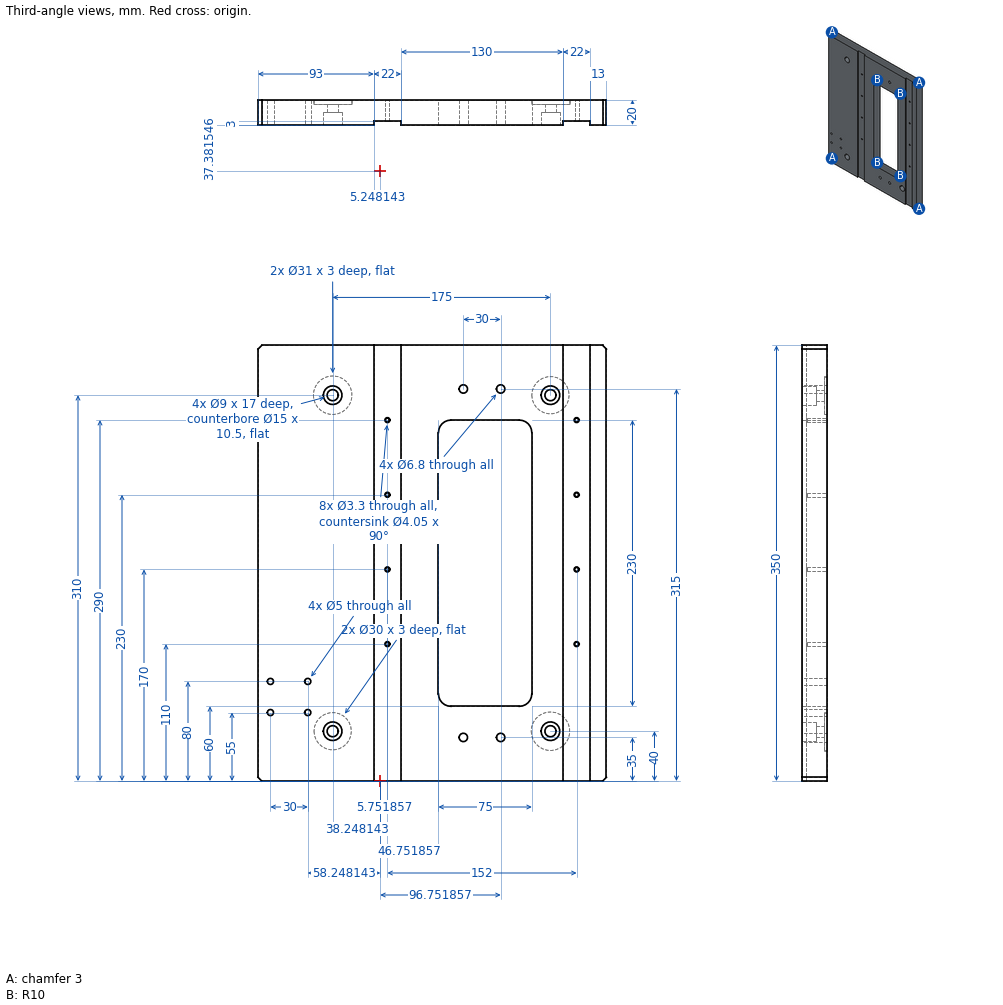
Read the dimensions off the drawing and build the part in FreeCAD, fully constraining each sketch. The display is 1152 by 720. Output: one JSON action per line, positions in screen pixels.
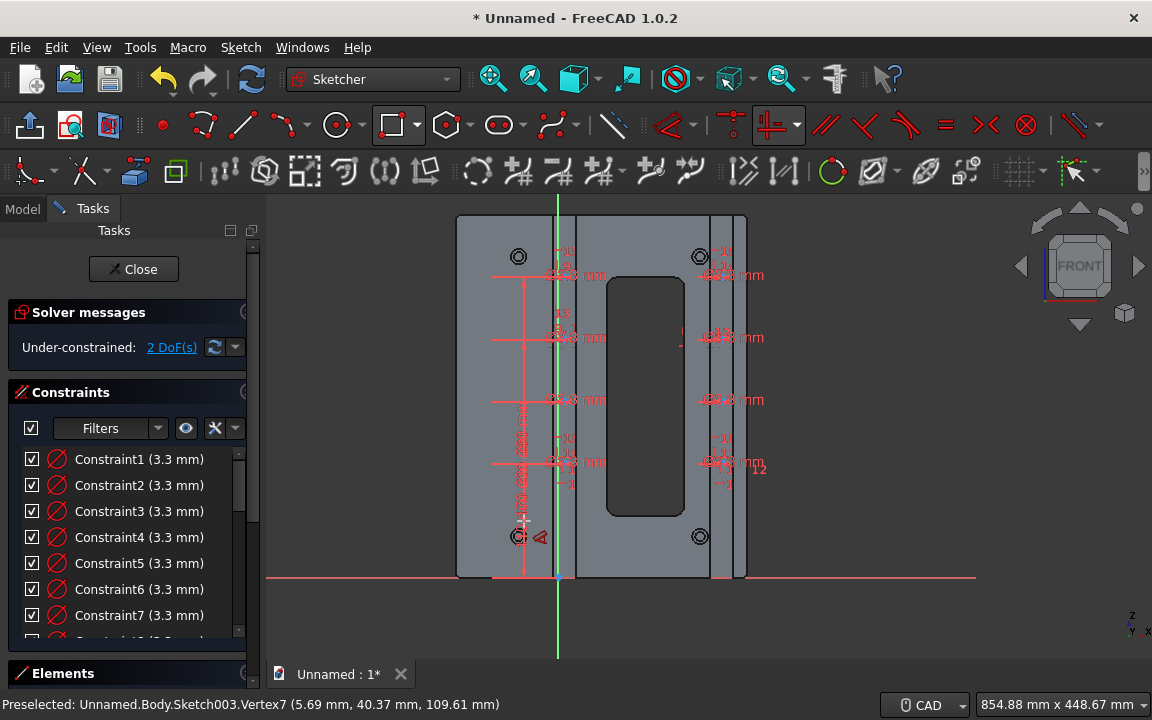
{"action": "left_click", "coordinate": [564, 402]}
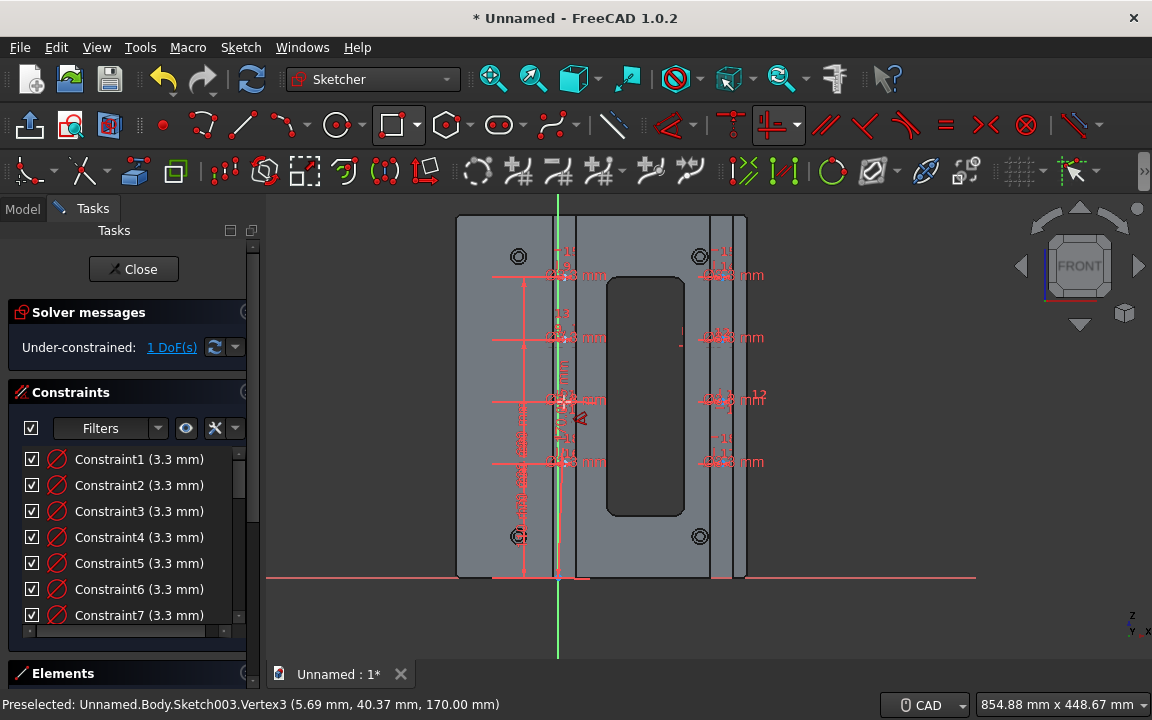
{"action": "left_click", "coordinate": [722, 402]}
{"action": "left_click", "coordinate": [643, 368]}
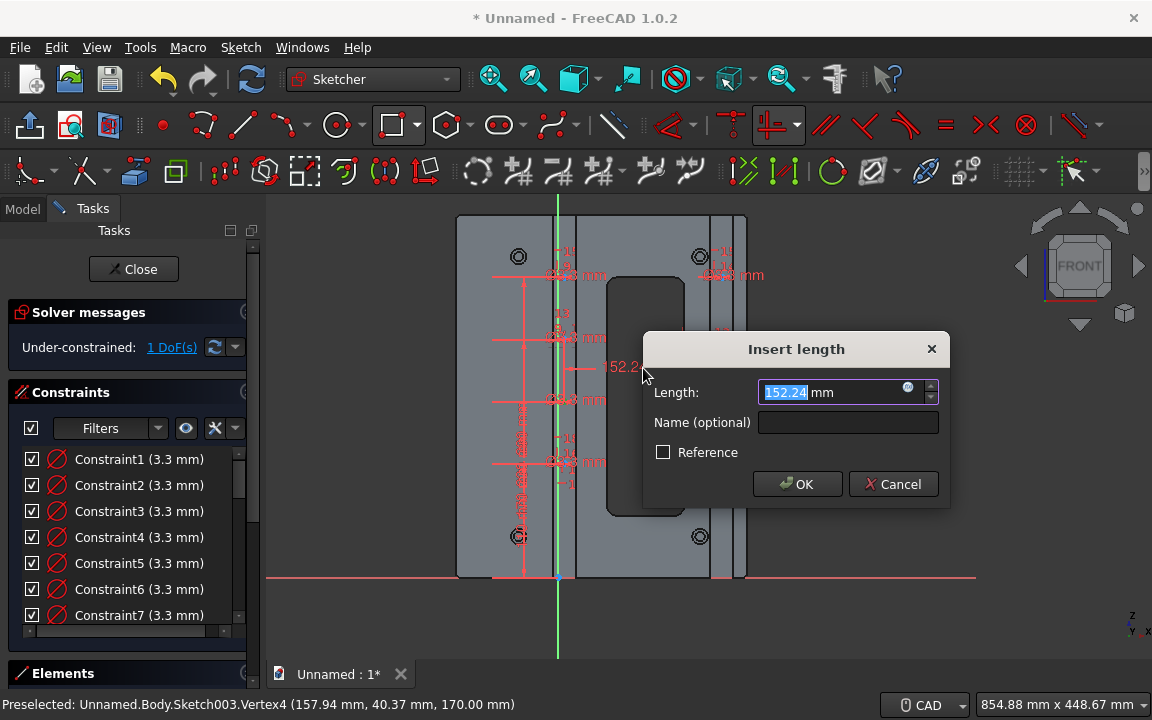
{"action": "type", "text": "152"}
{"action": "key", "text": "Return"}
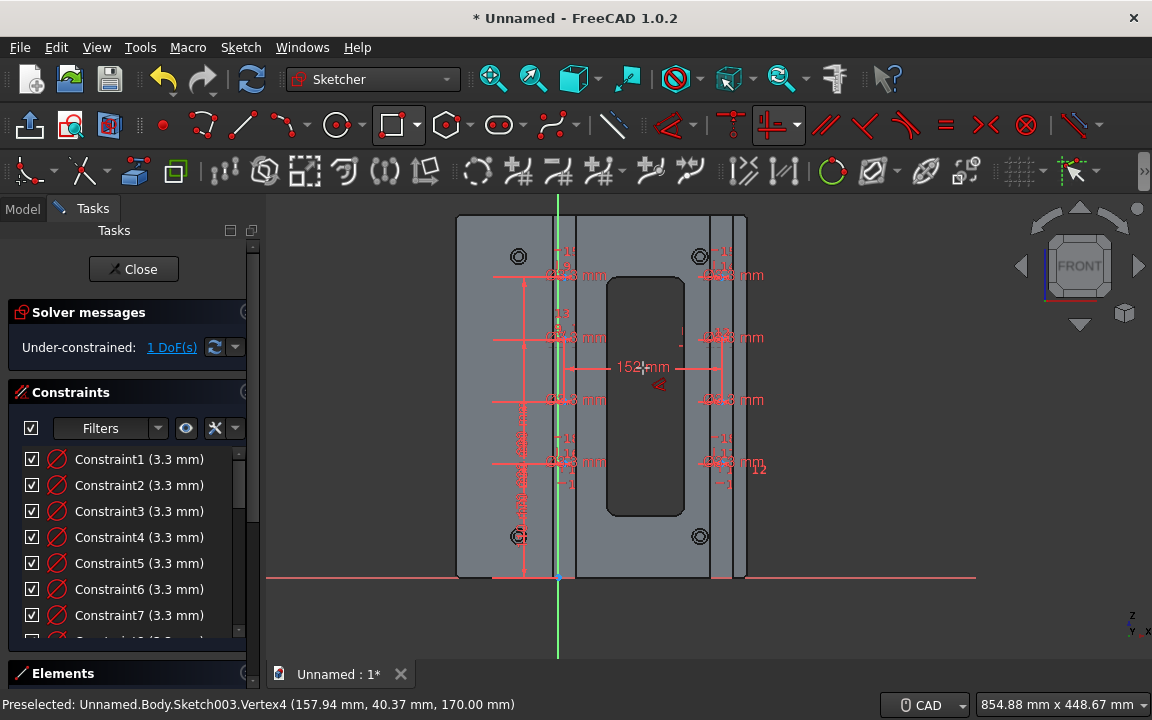
{"action": "scroll", "coordinate": [564, 277], "scroll_direction": "up", "scroll_amount": 10}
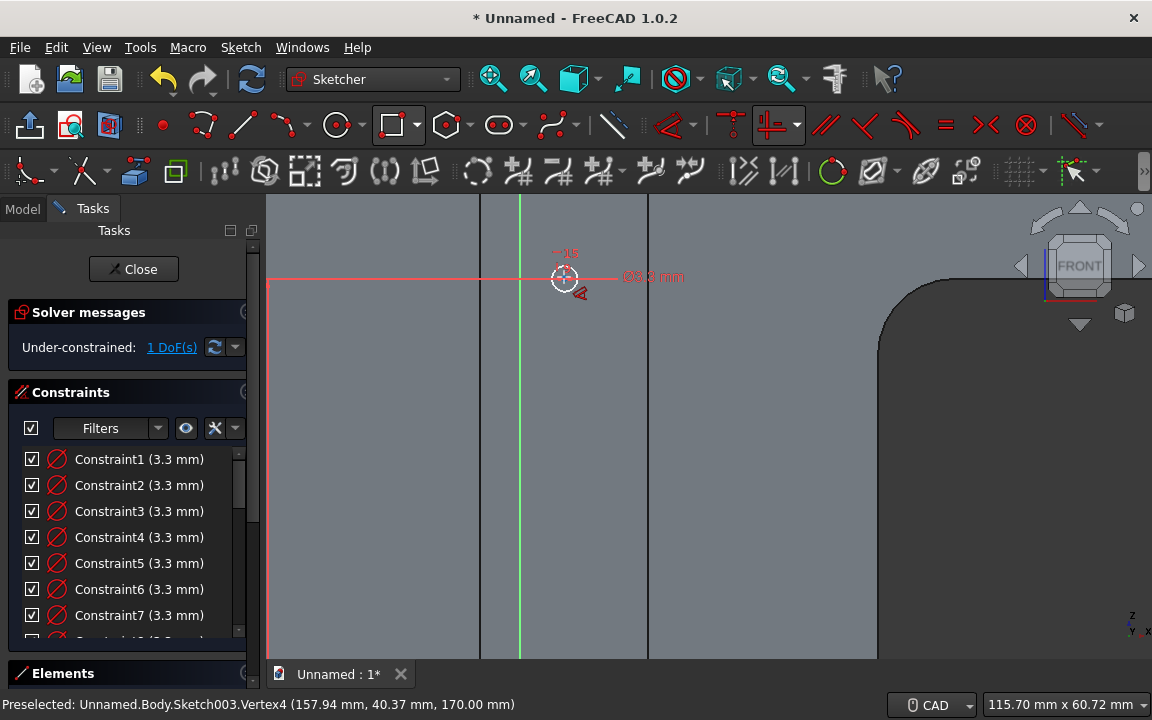
{"action": "left_click", "coordinate": [565, 279]}
{"action": "left_click", "coordinate": [542, 245]}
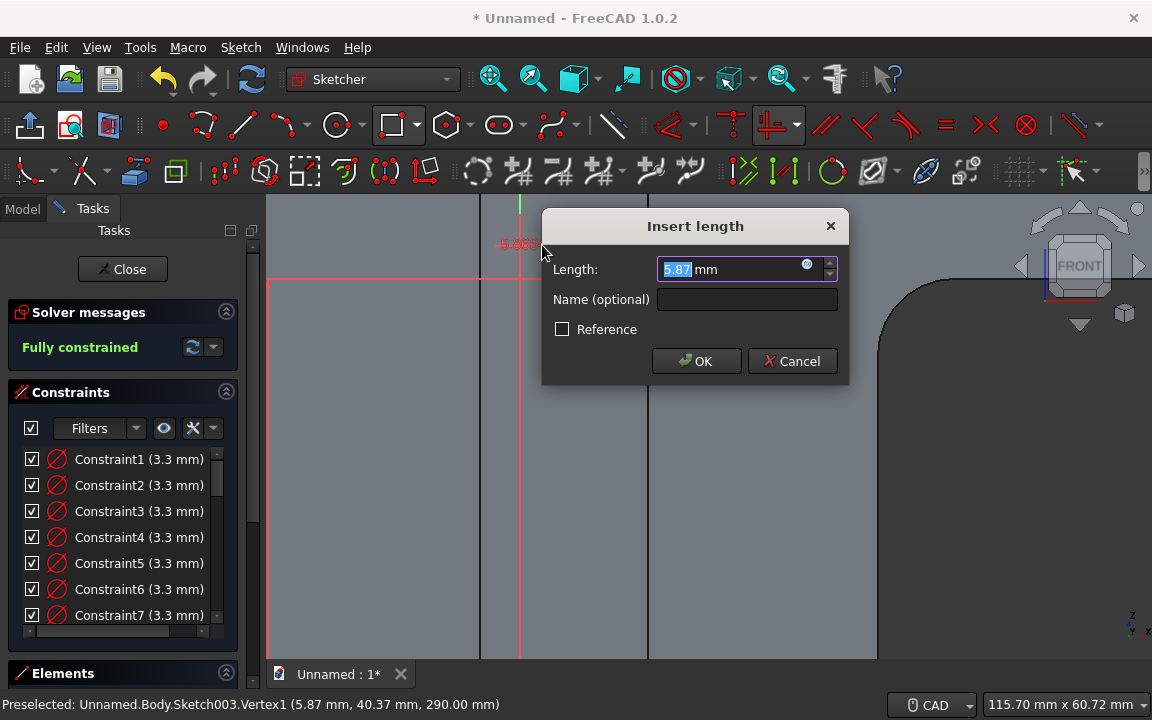
{"action": "type", "text": "5.751857"}
{"action": "key", "text": "Return"}
{"action": "key", "text": "Escape"}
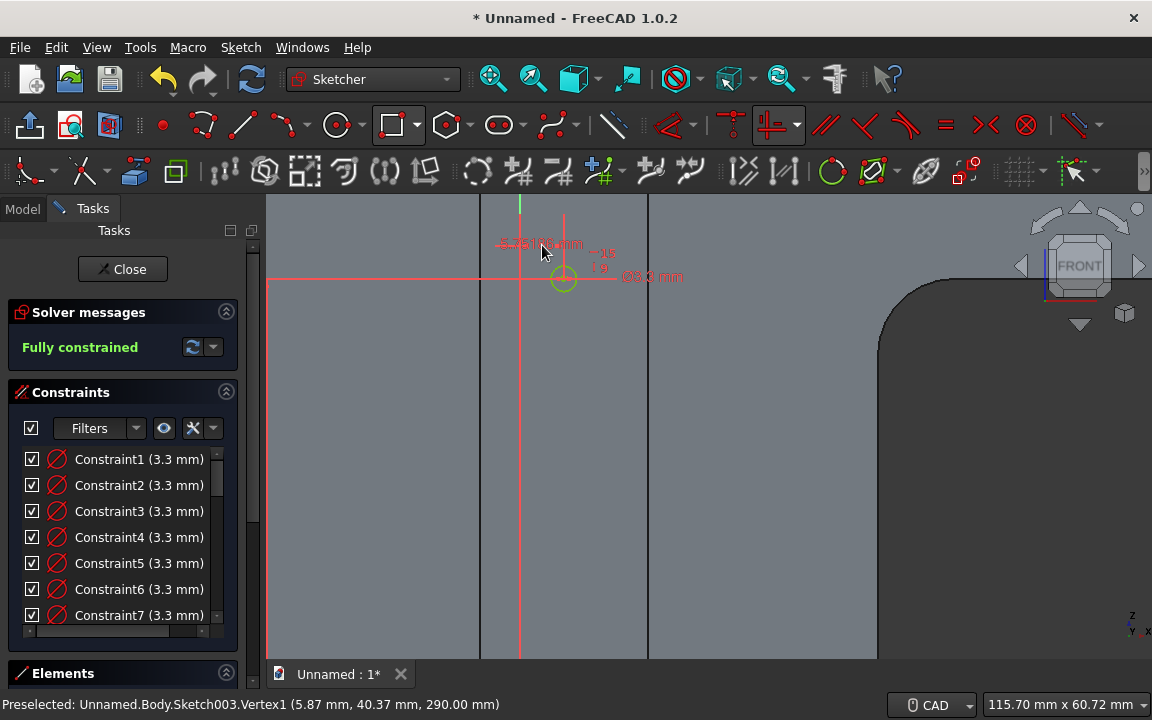
{"action": "left_click", "coordinate": [123, 269]}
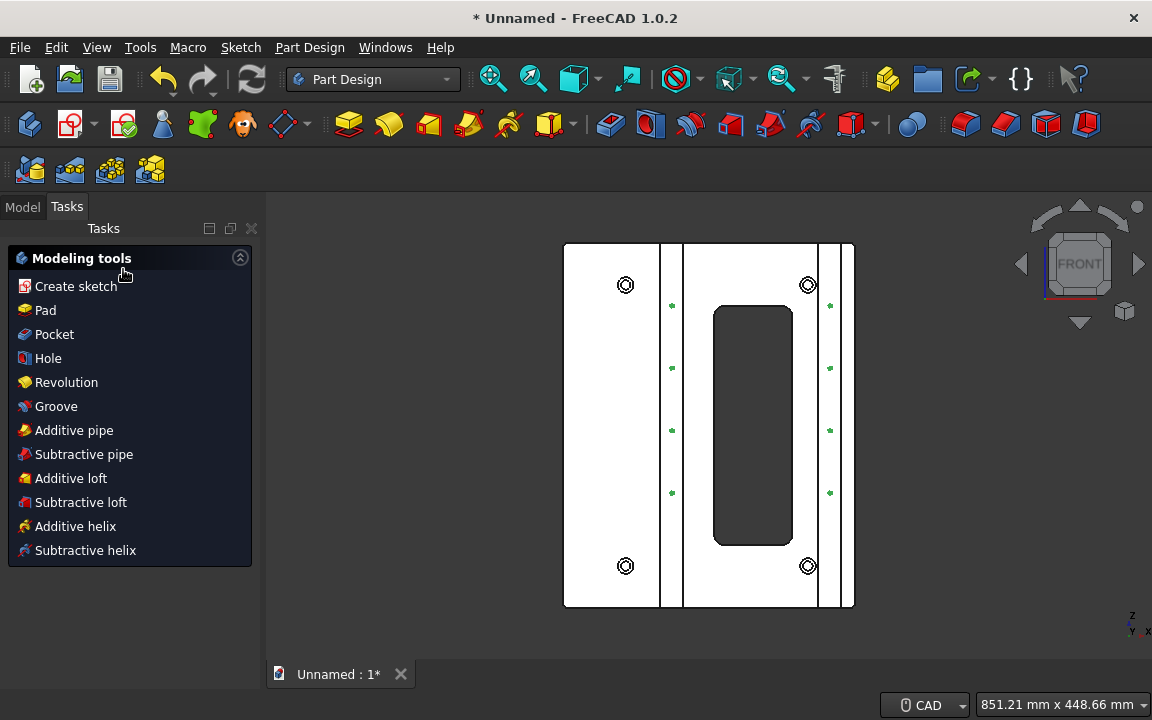
{"action": "left_click", "coordinate": [652, 124]}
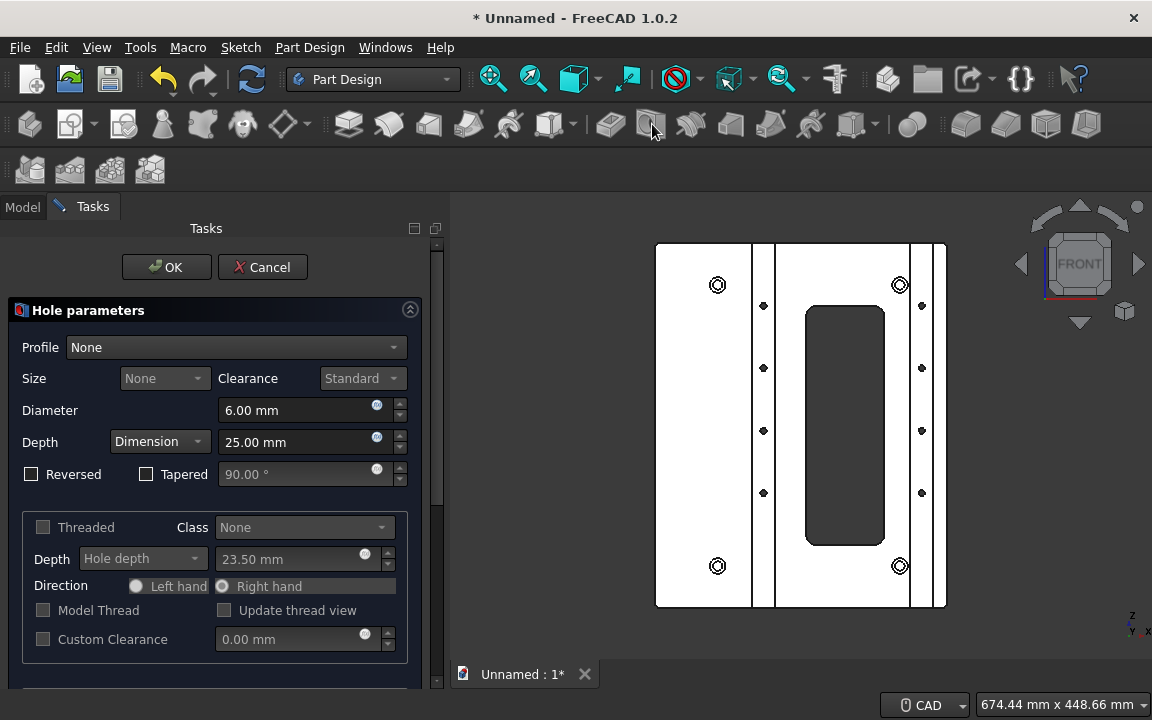
{"action": "triple_click", "coordinate": [305, 410]}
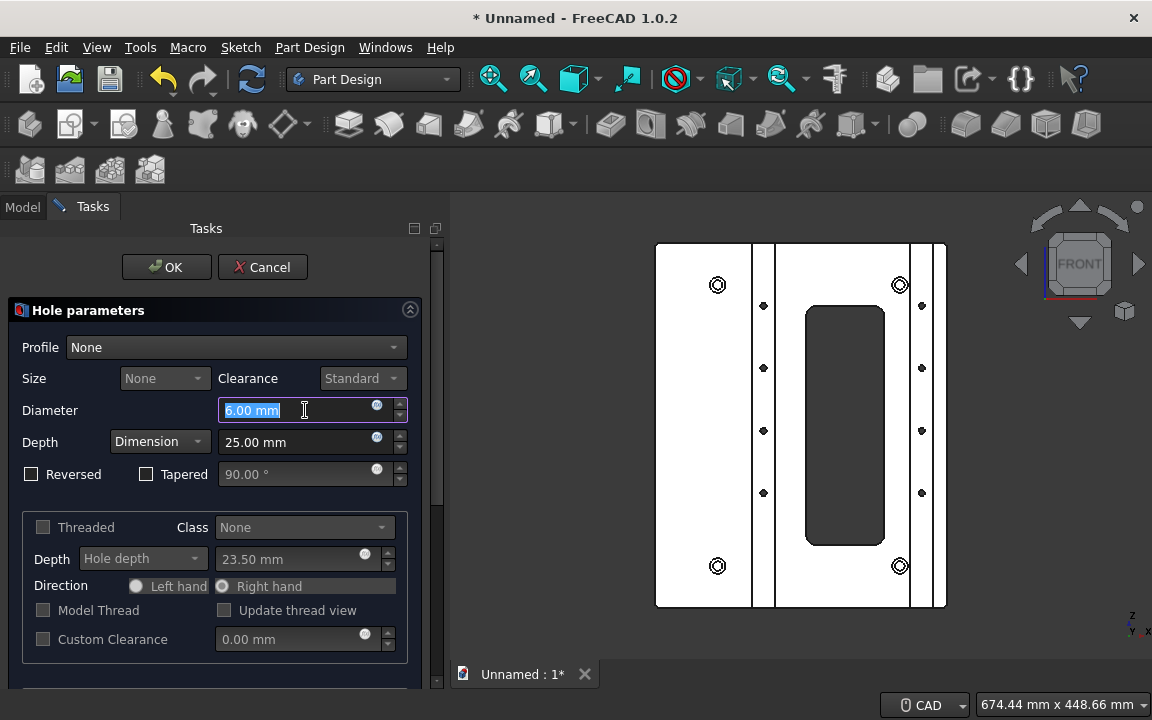
{"action": "type", "text": "3.3"}
{"action": "key", "text": "Tab"}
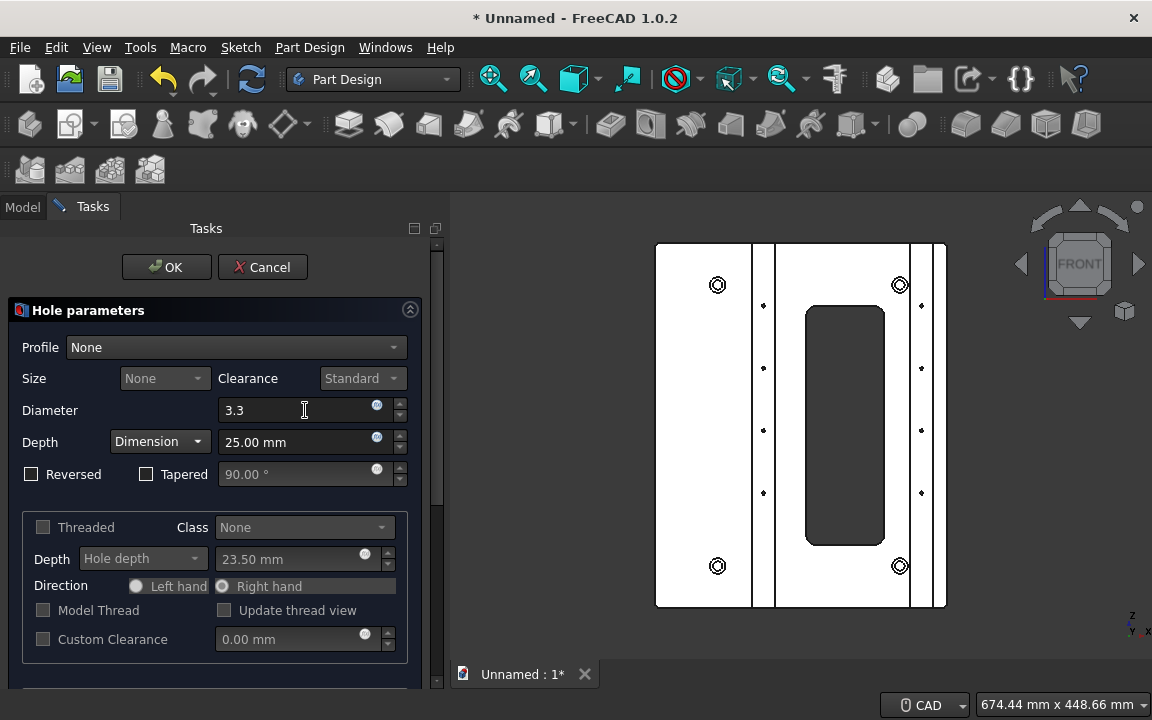
{"action": "left_click", "coordinate": [161, 442]}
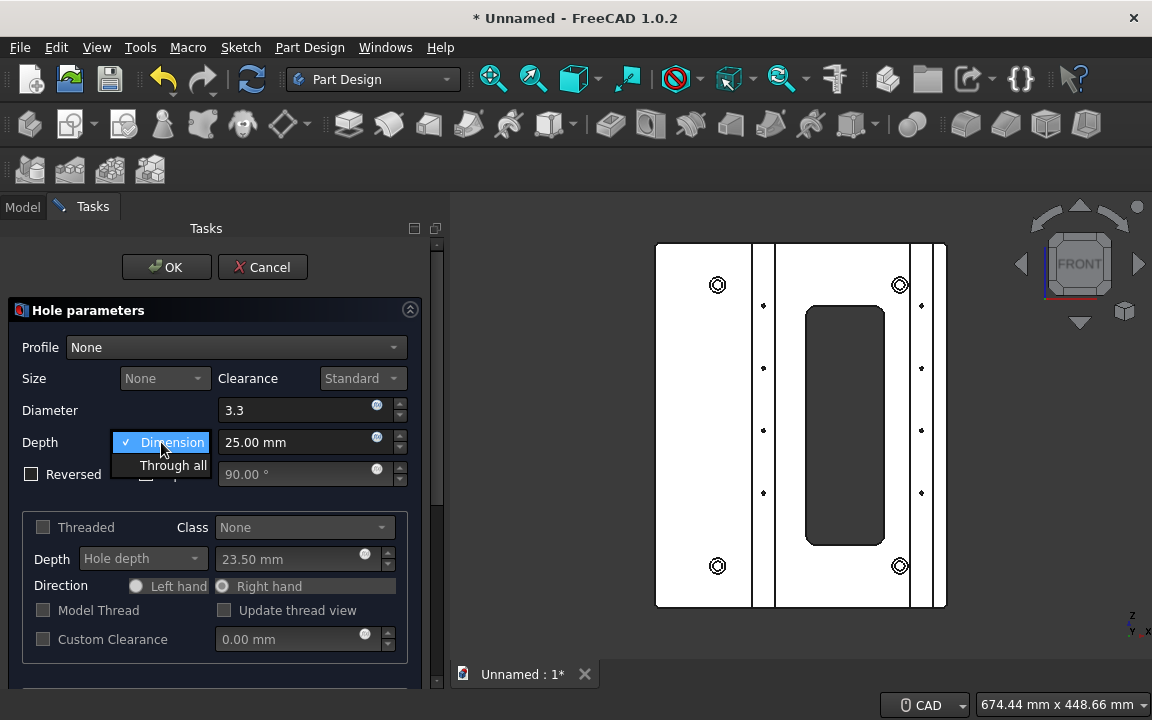
{"action": "left_click", "coordinate": [160, 466]}